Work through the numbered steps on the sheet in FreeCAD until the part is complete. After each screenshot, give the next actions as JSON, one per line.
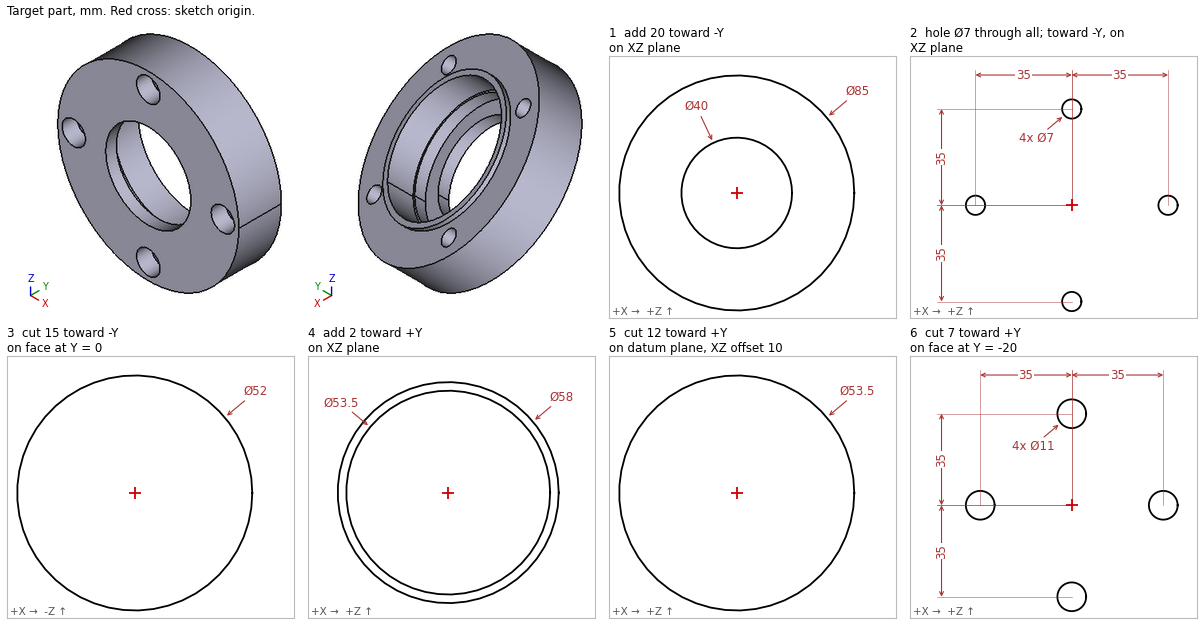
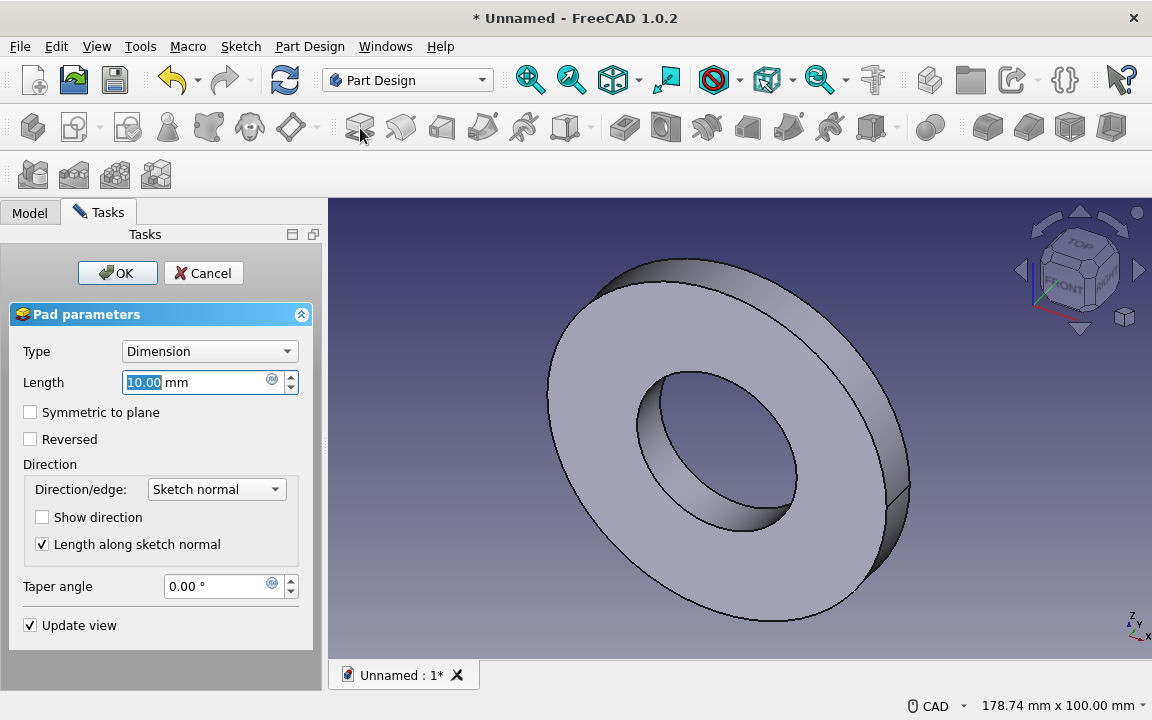
{"action": "type", "text": "20"}
{"action": "key", "text": "Tab"}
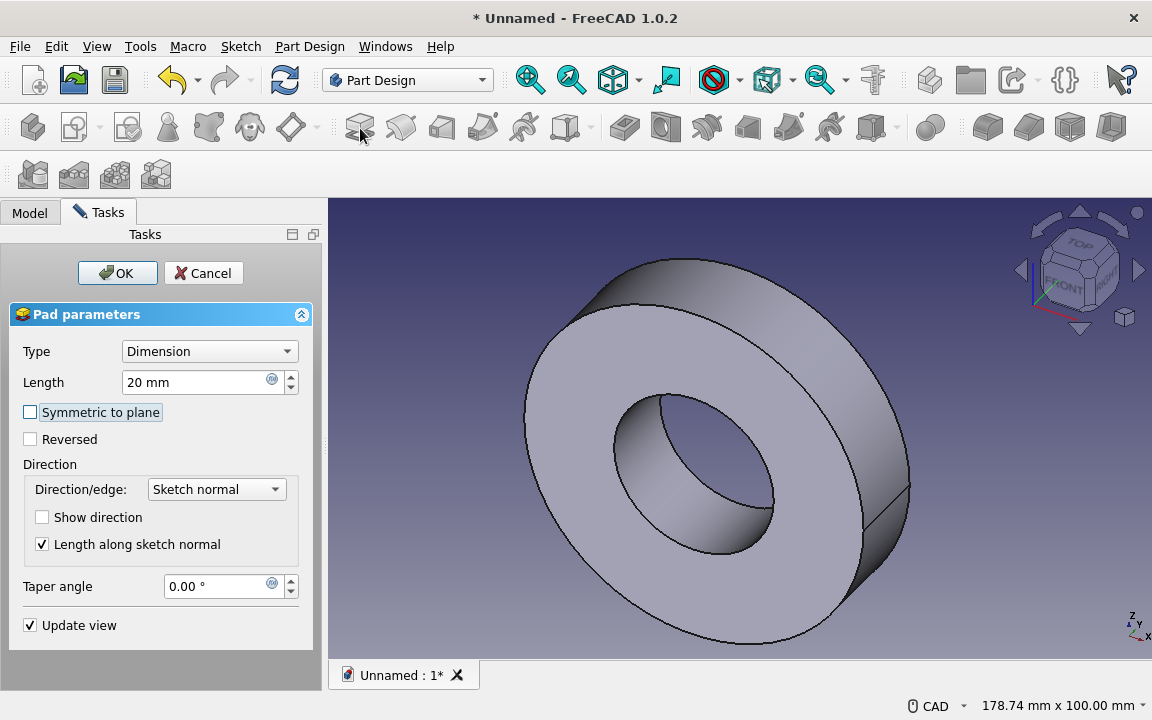
{"action": "left_click", "coordinate": [118, 273]}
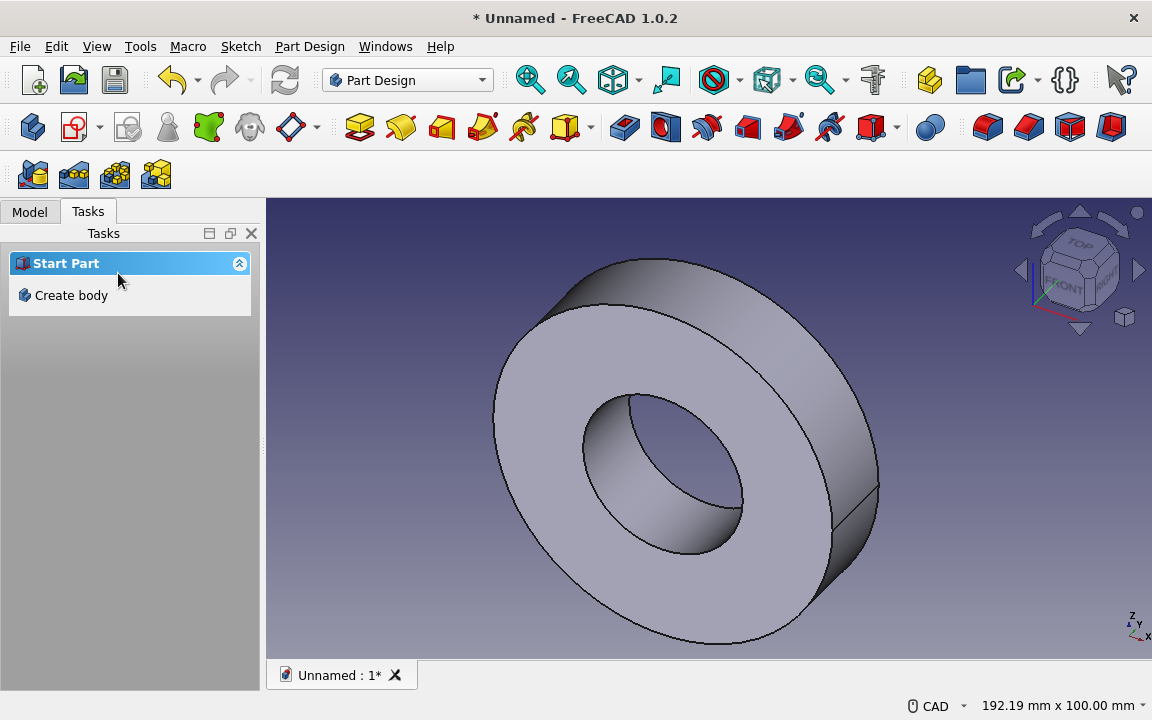
{"action": "left_click", "coordinate": [531, 80]}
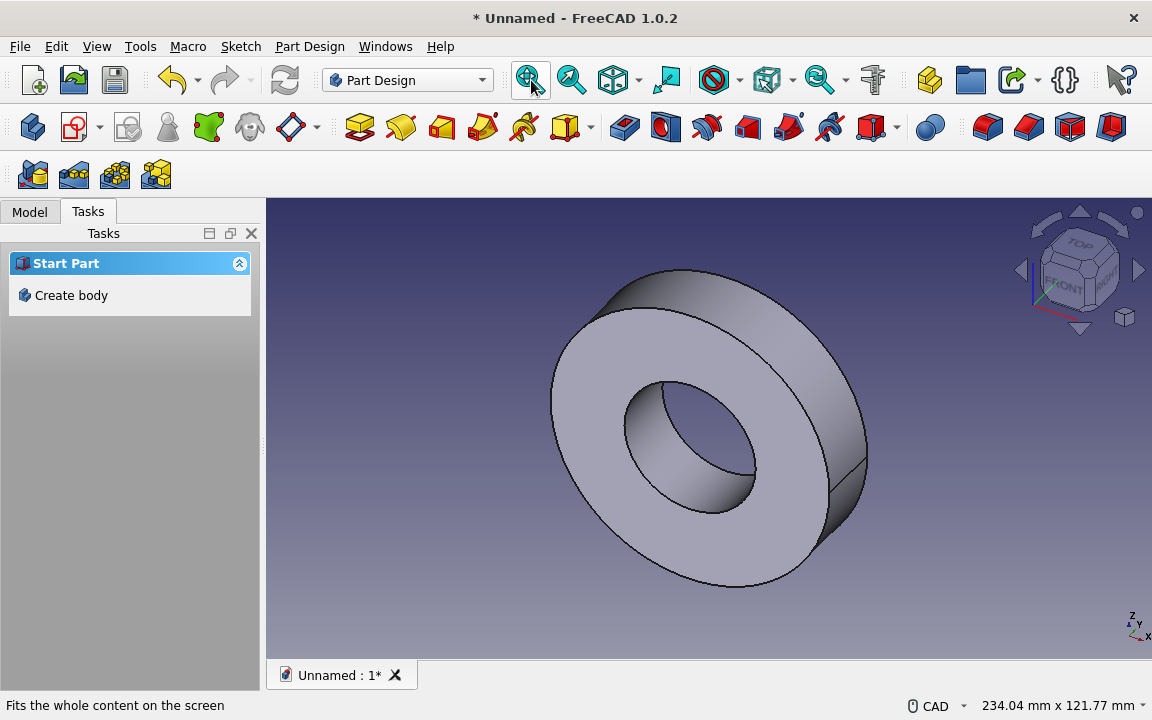
{"action": "left_click", "coordinate": [74, 128]}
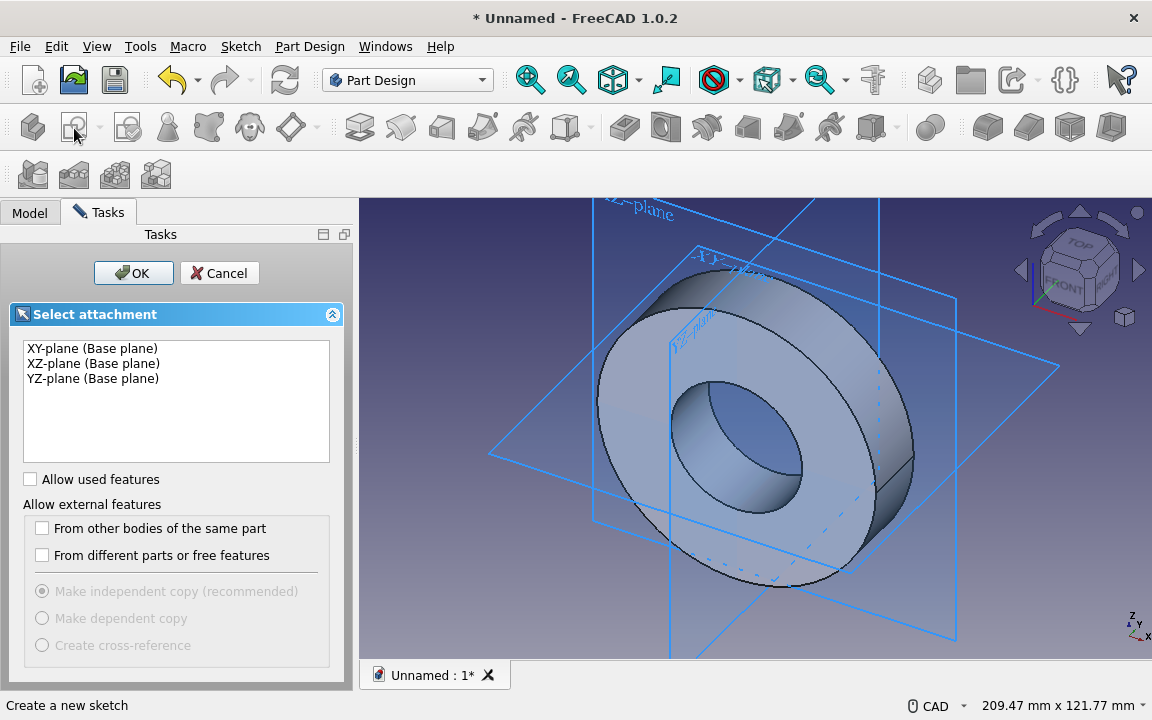
{"action": "left_click", "coordinate": [84, 364]}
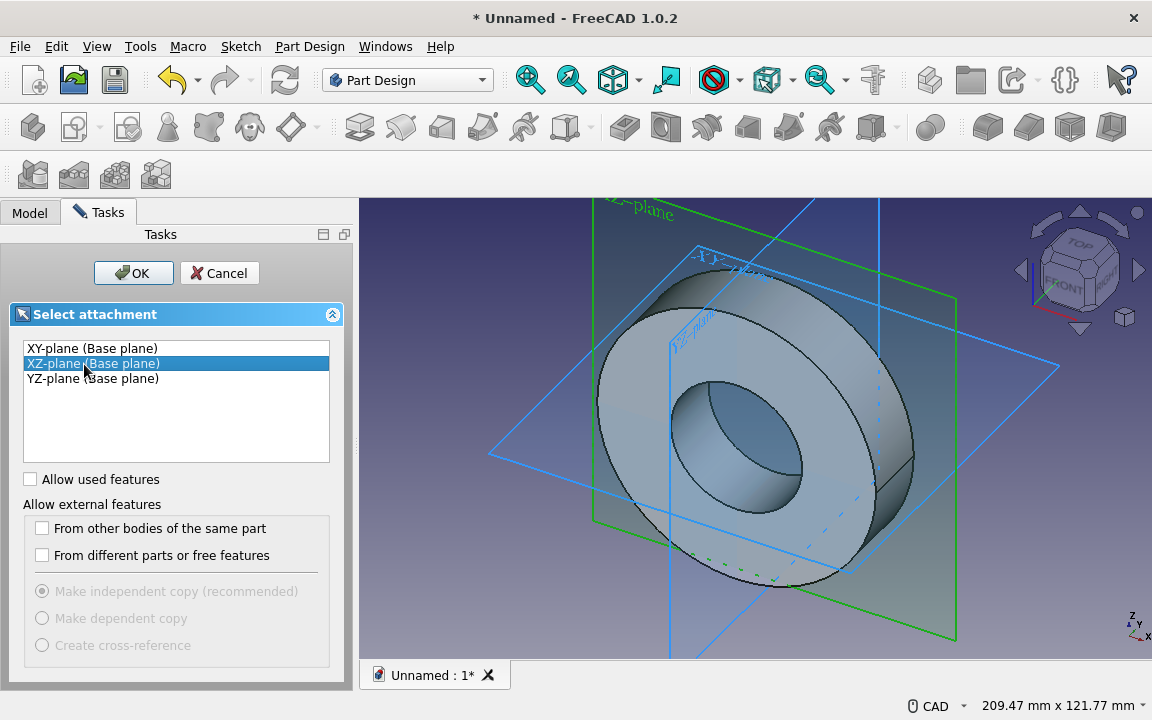
{"action": "left_click", "coordinate": [134, 273]}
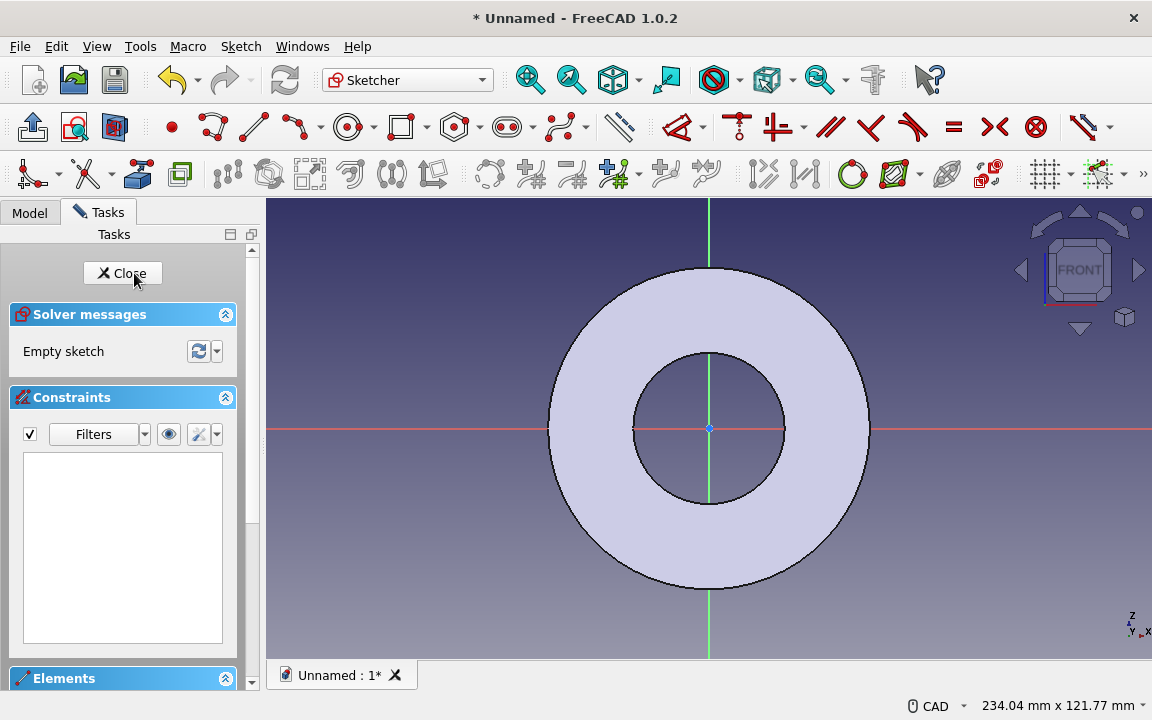
{"action": "key", "text": "q s"}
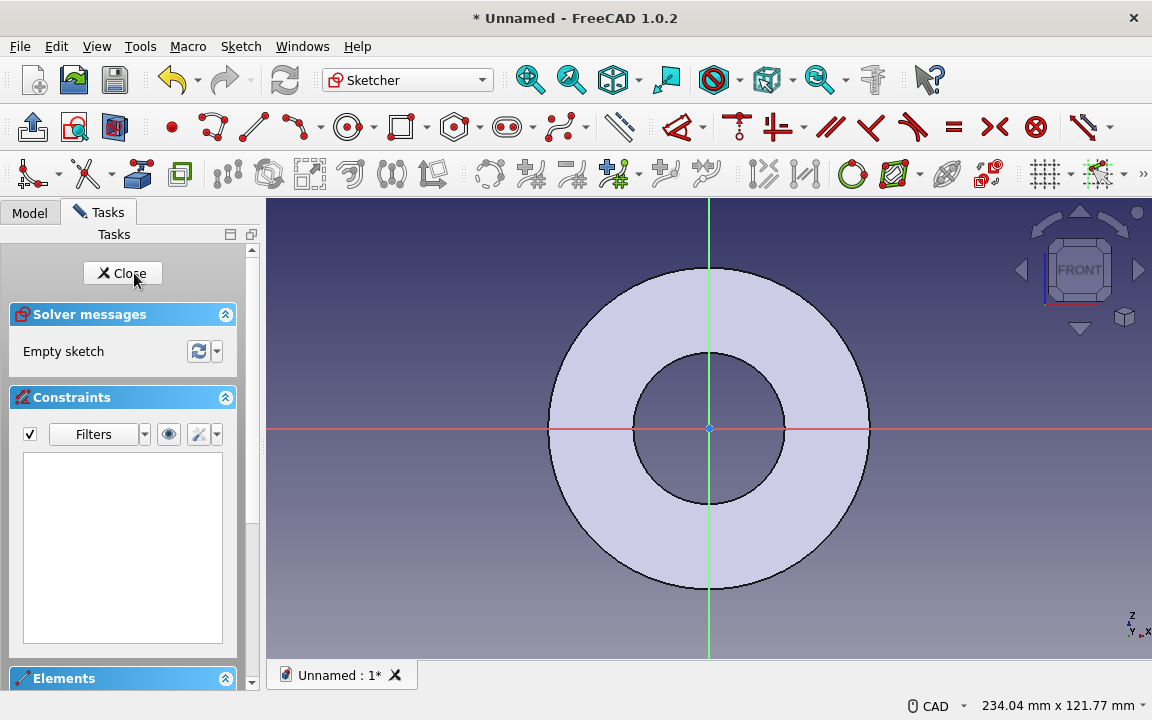
{"action": "key", "text": "g c"}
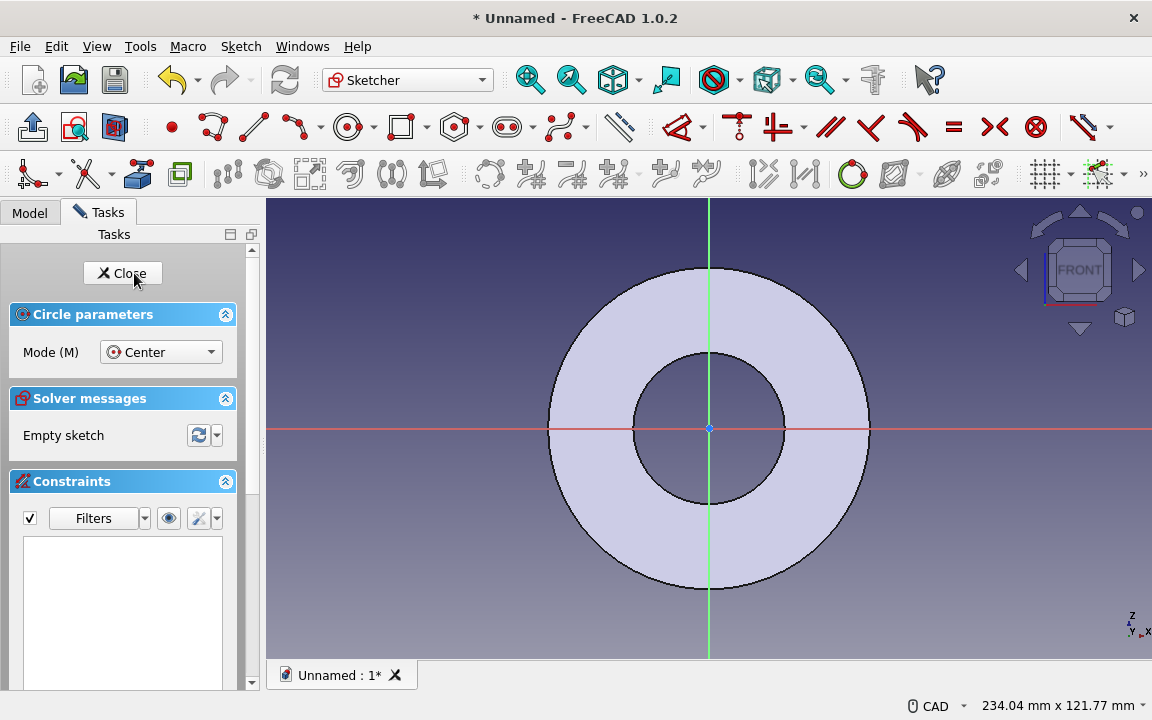
{"action": "scroll", "coordinate": [709, 296], "scroll_direction": "up", "scroll_amount": 3}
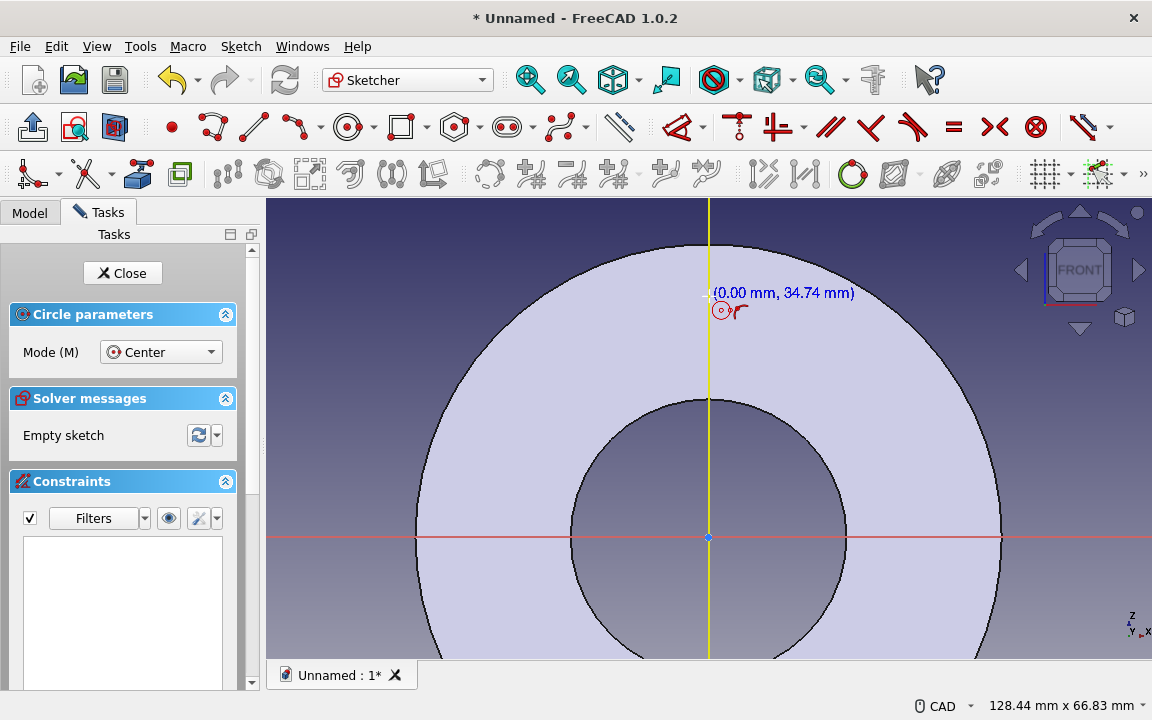
{"action": "left_click", "coordinate": [709, 296]}
{"action": "mouse_move", "coordinate": [726, 279]}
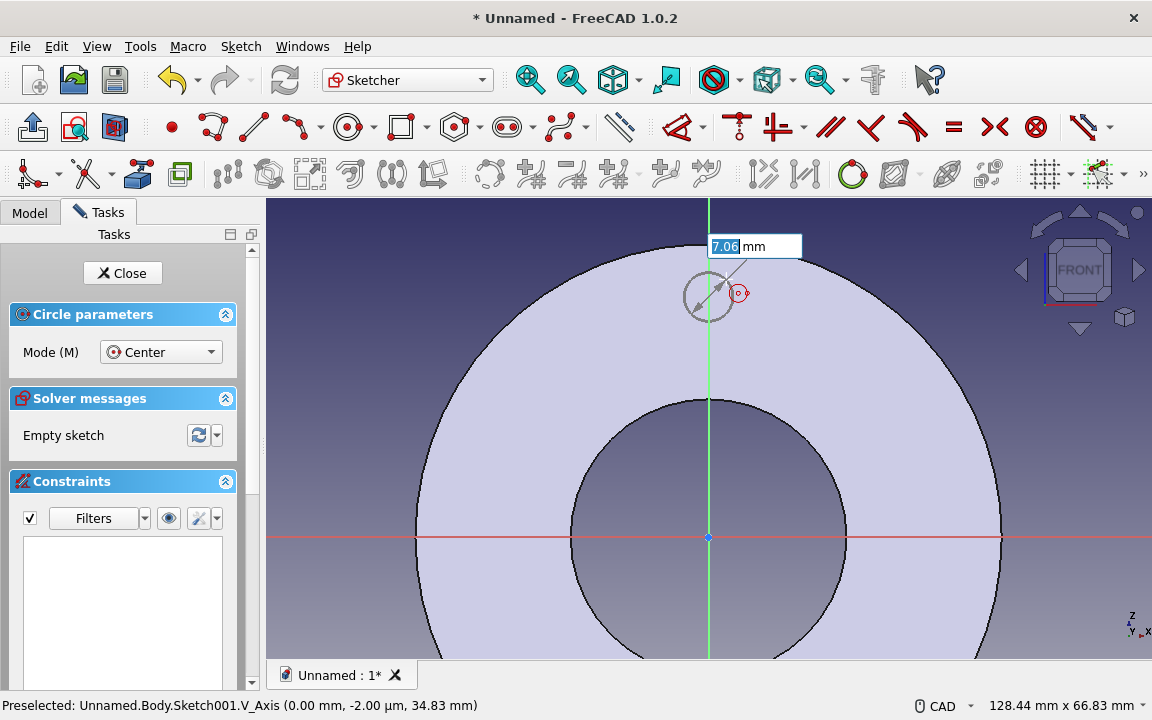
{"action": "type", "text": "7"}
{"action": "key", "text": "Return"}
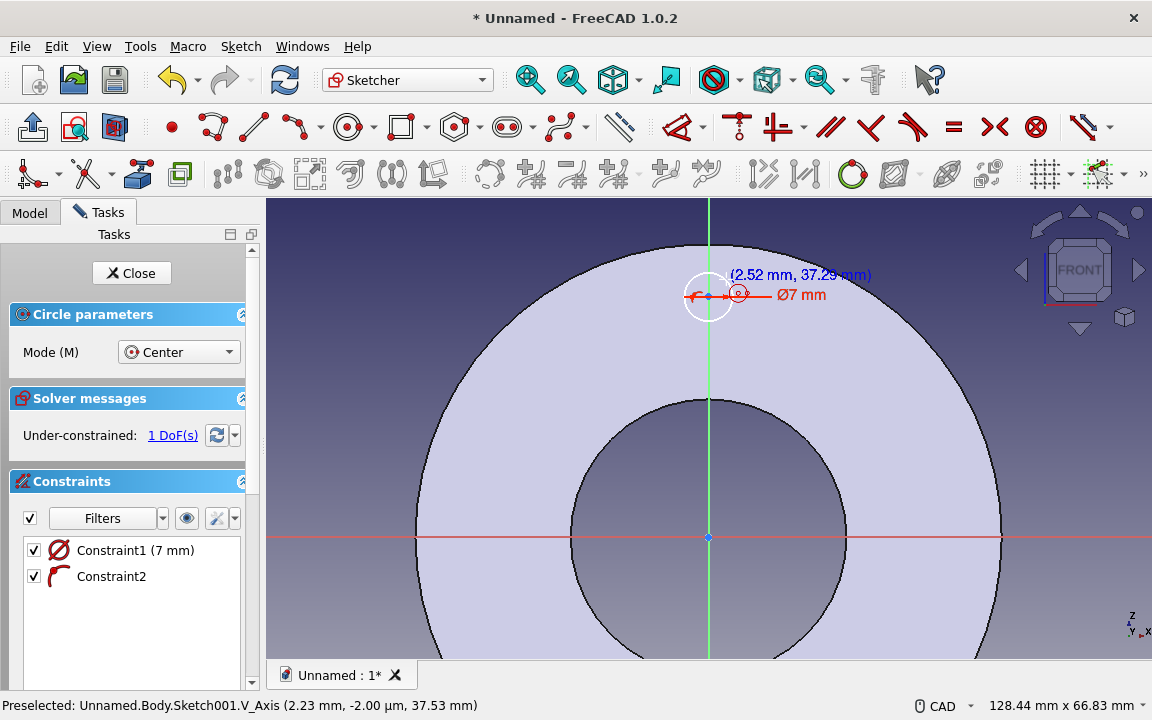
{"action": "scroll", "coordinate": [558, 296], "scroll_direction": "down", "scroll_amount": 3}